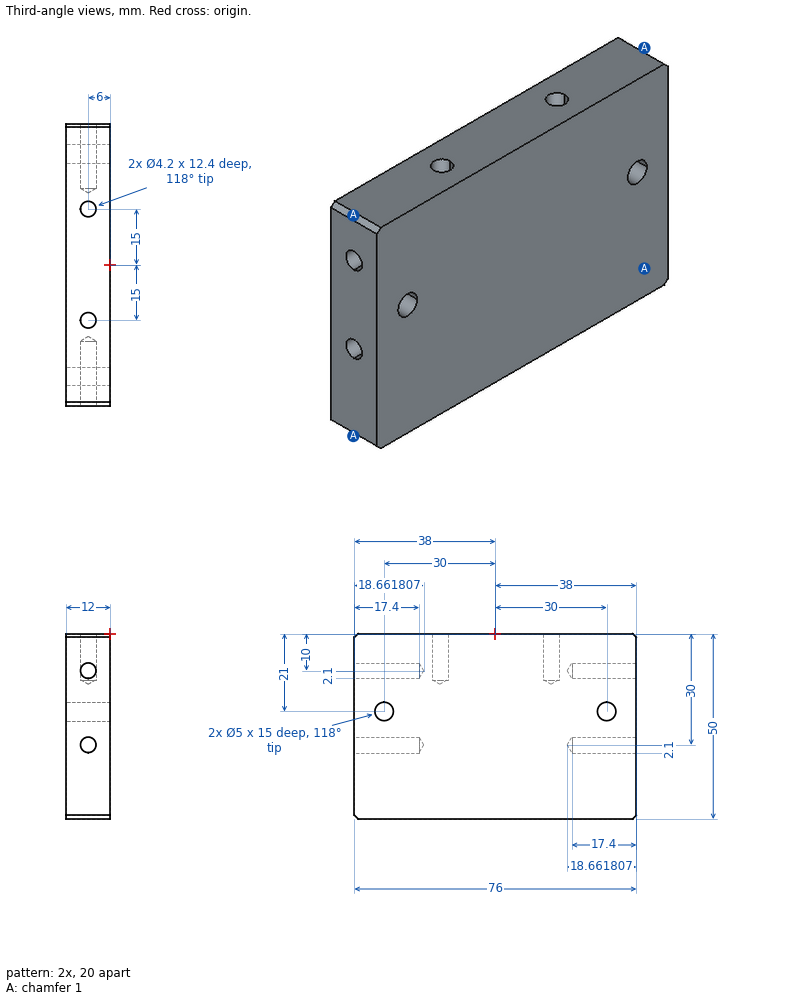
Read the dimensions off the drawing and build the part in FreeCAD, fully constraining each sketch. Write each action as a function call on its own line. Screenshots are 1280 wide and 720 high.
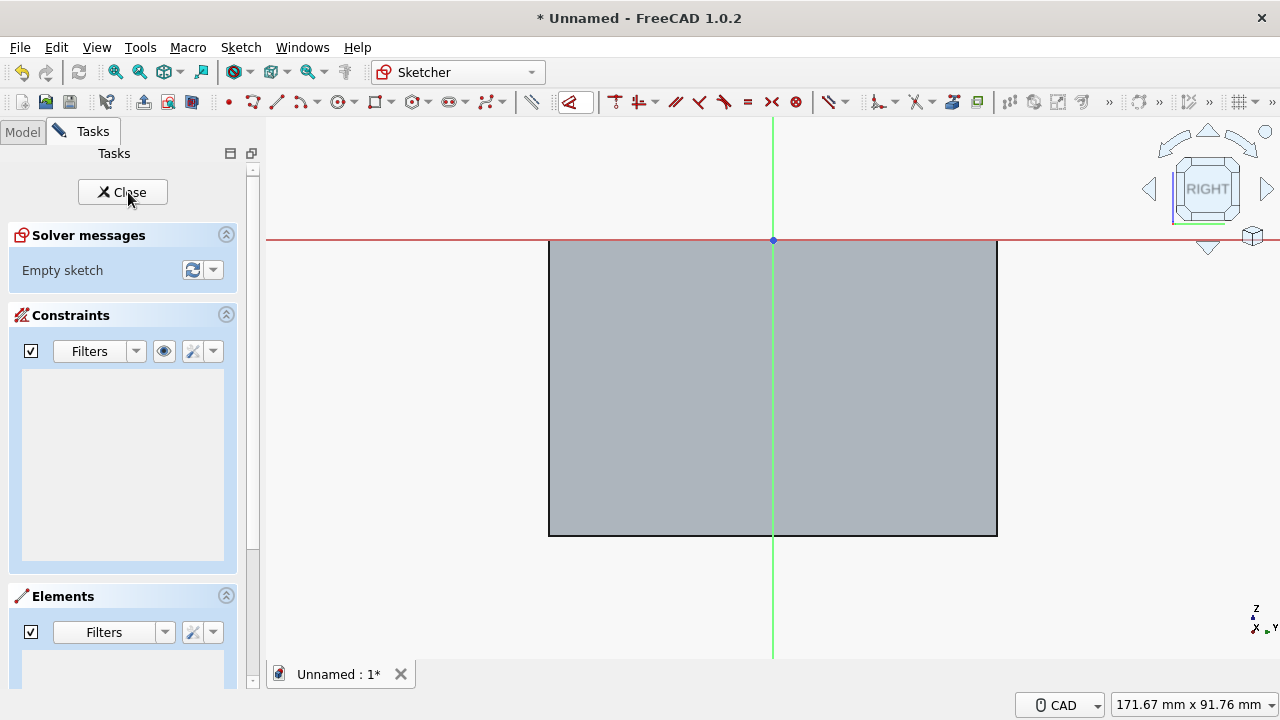
scroll(912, 151, up, 2)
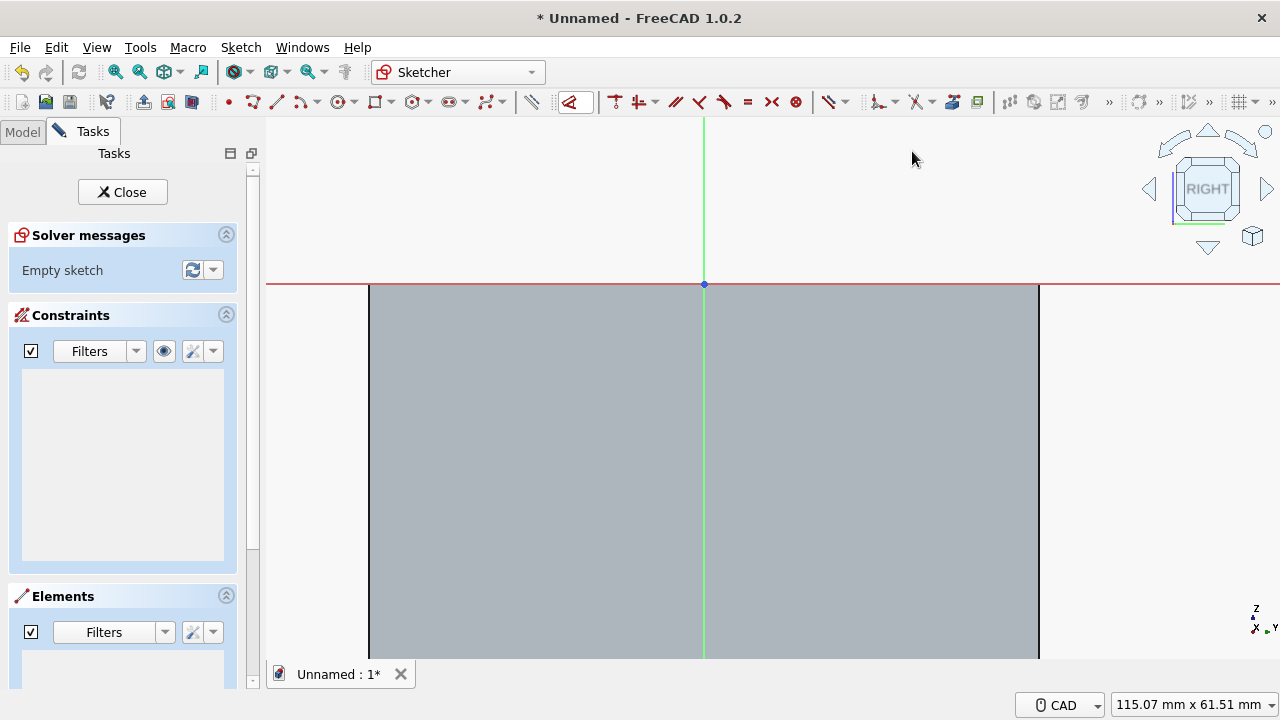
click(338, 102)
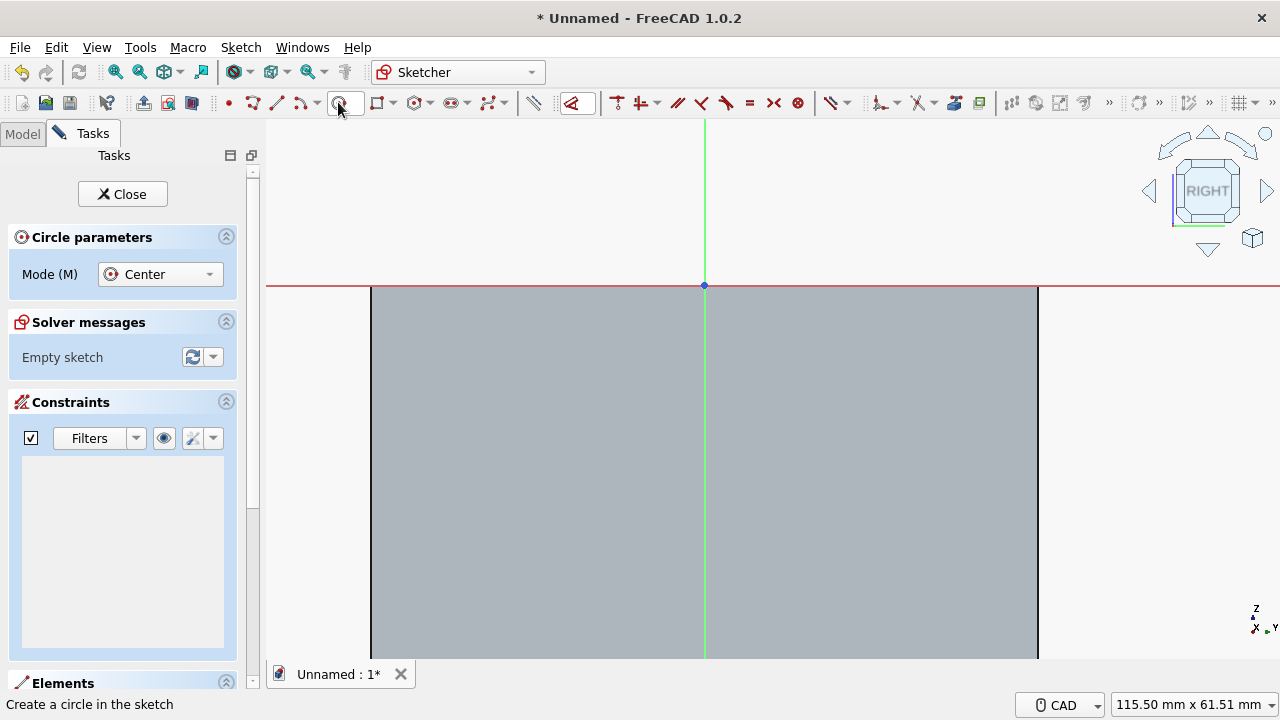
click(441, 470)
move(457, 454)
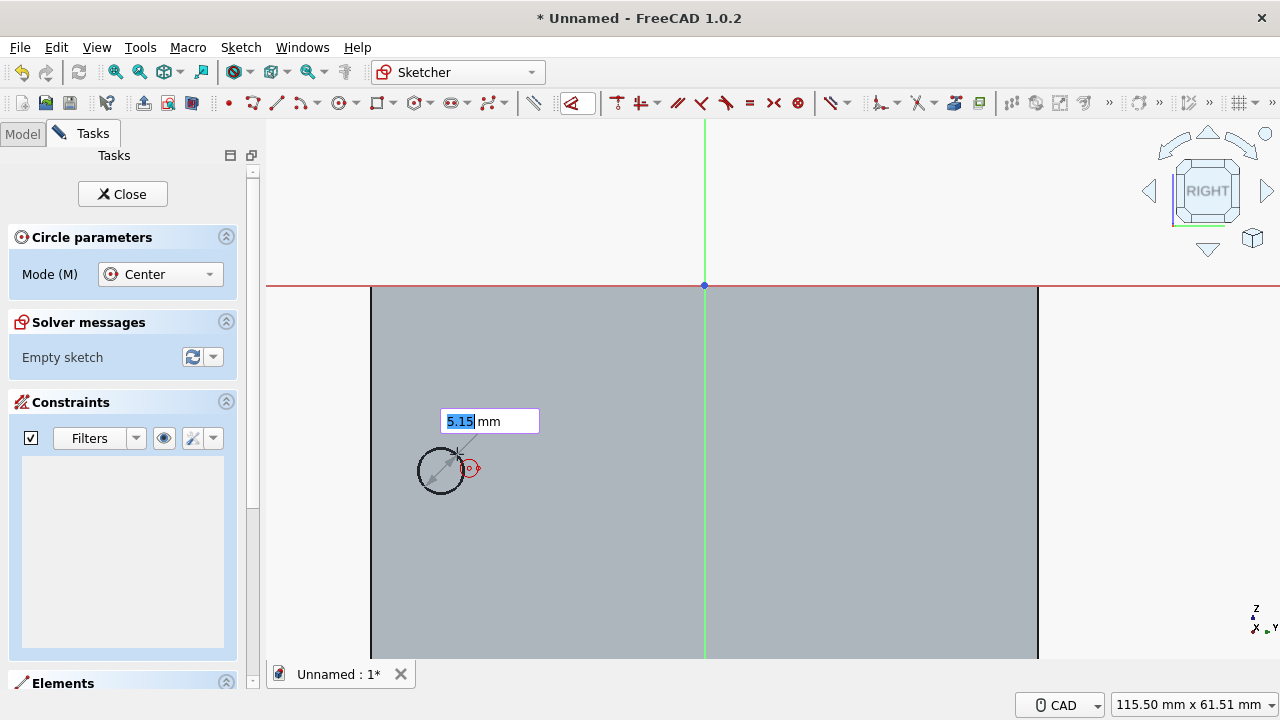
text(5)
key(Return)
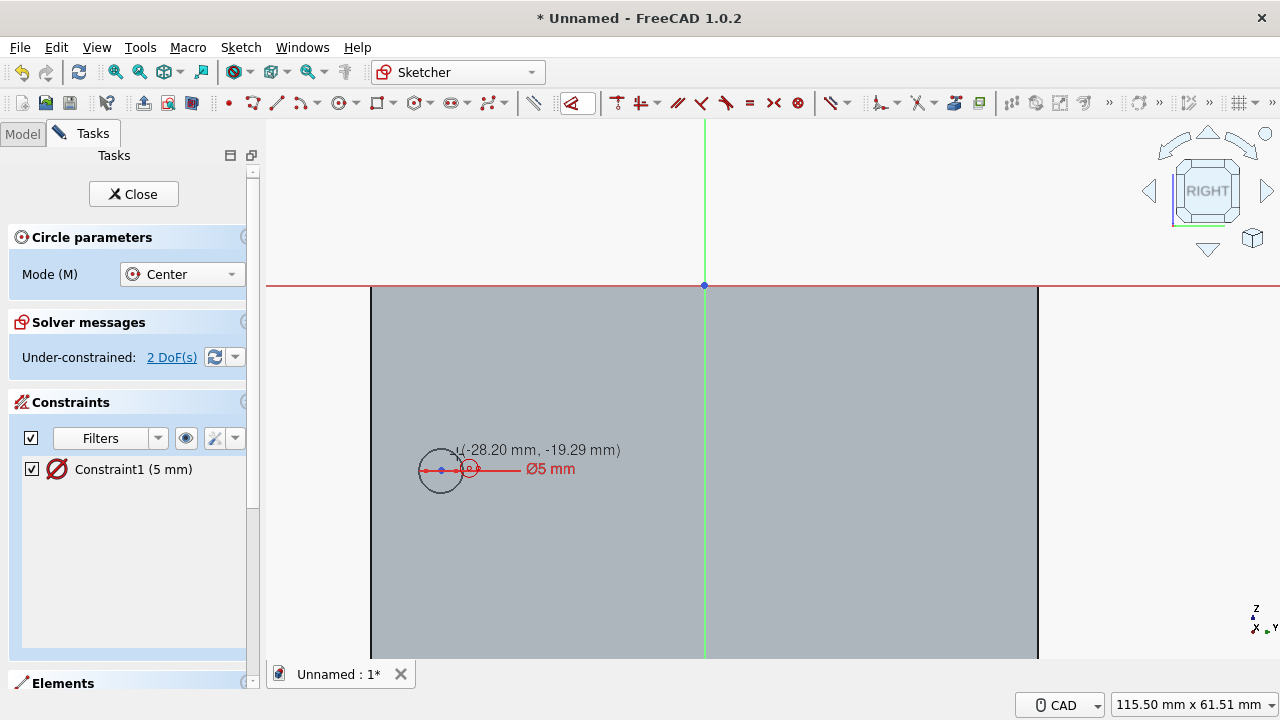
click(968, 470)
move(983, 454)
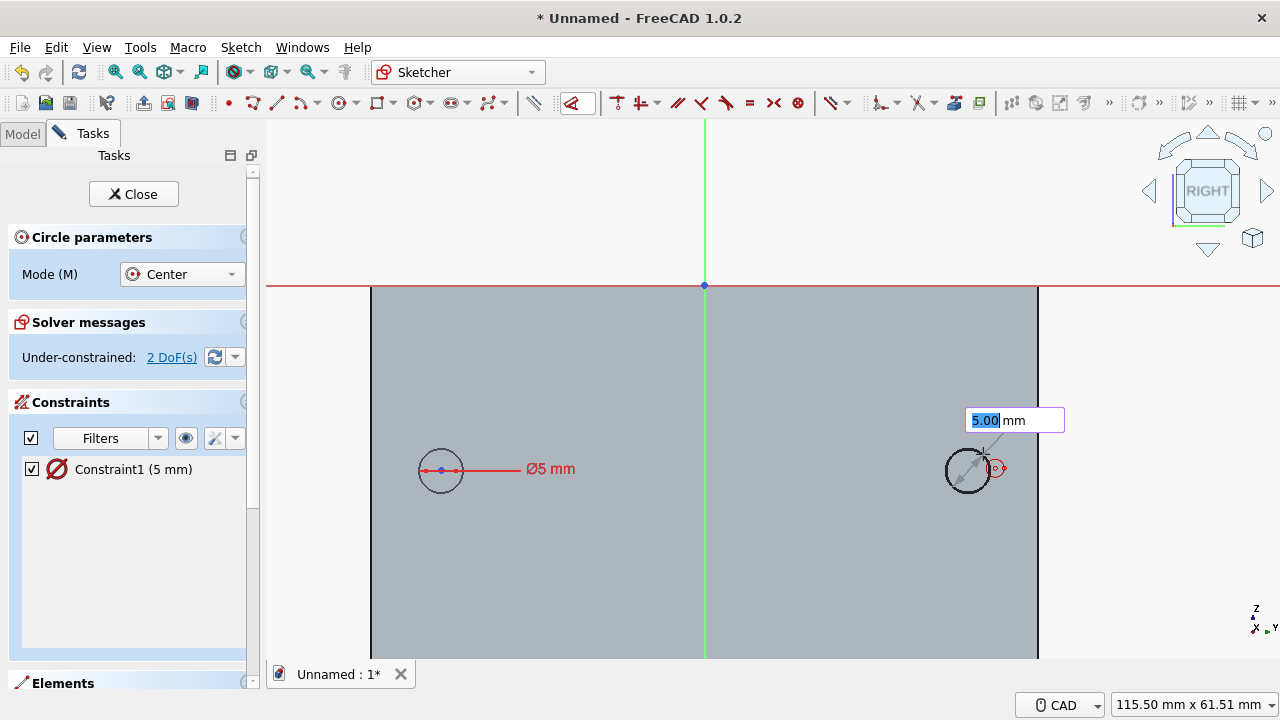
text(5)
key(Return)
key(Escape)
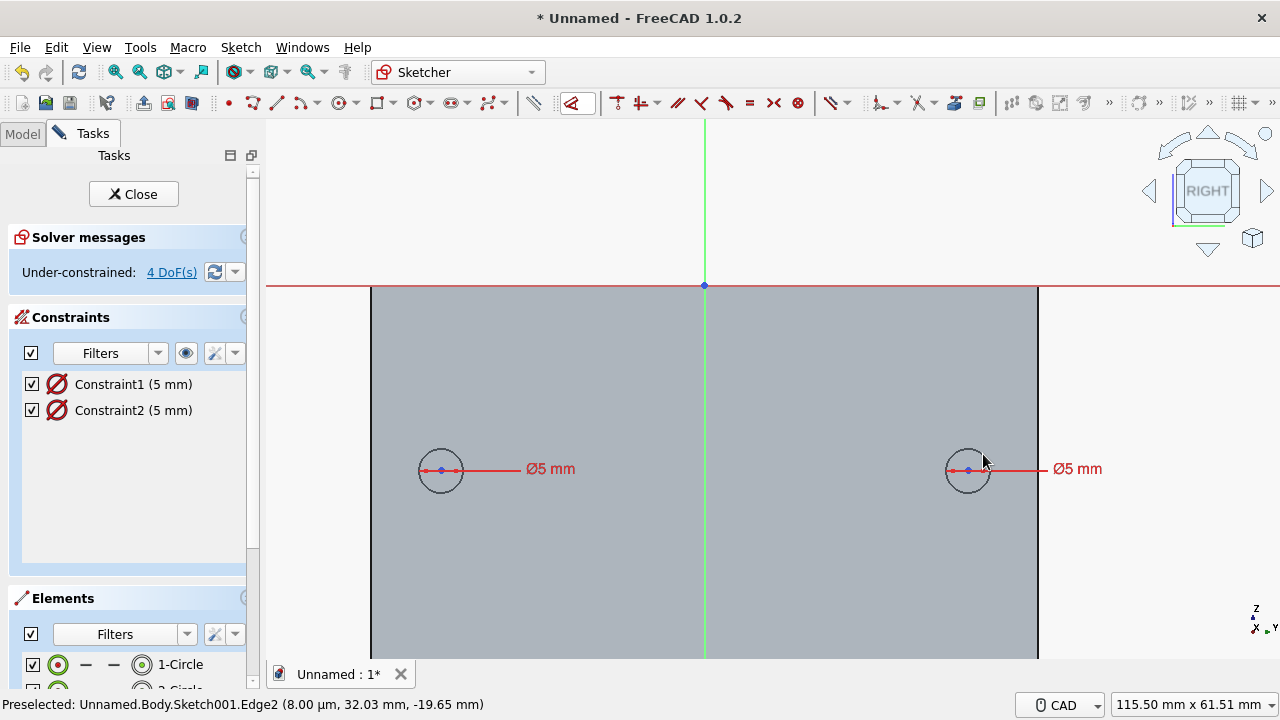
click(441, 471)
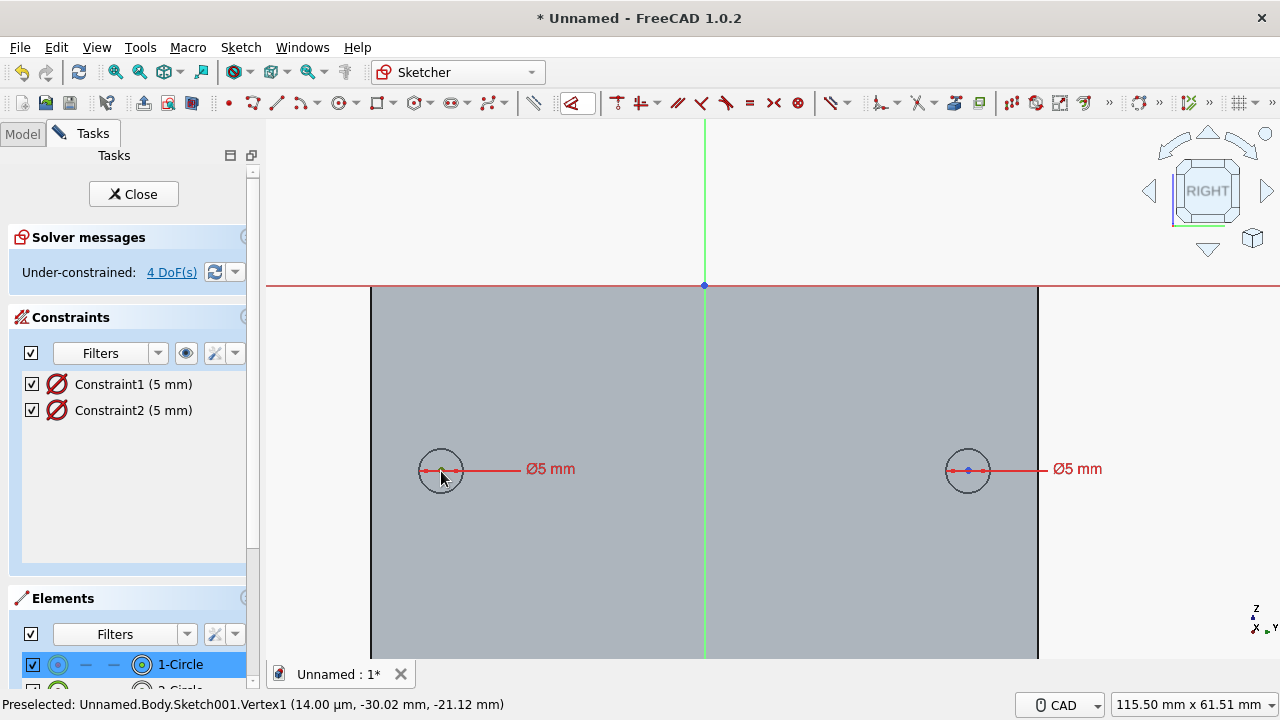
click(968, 471)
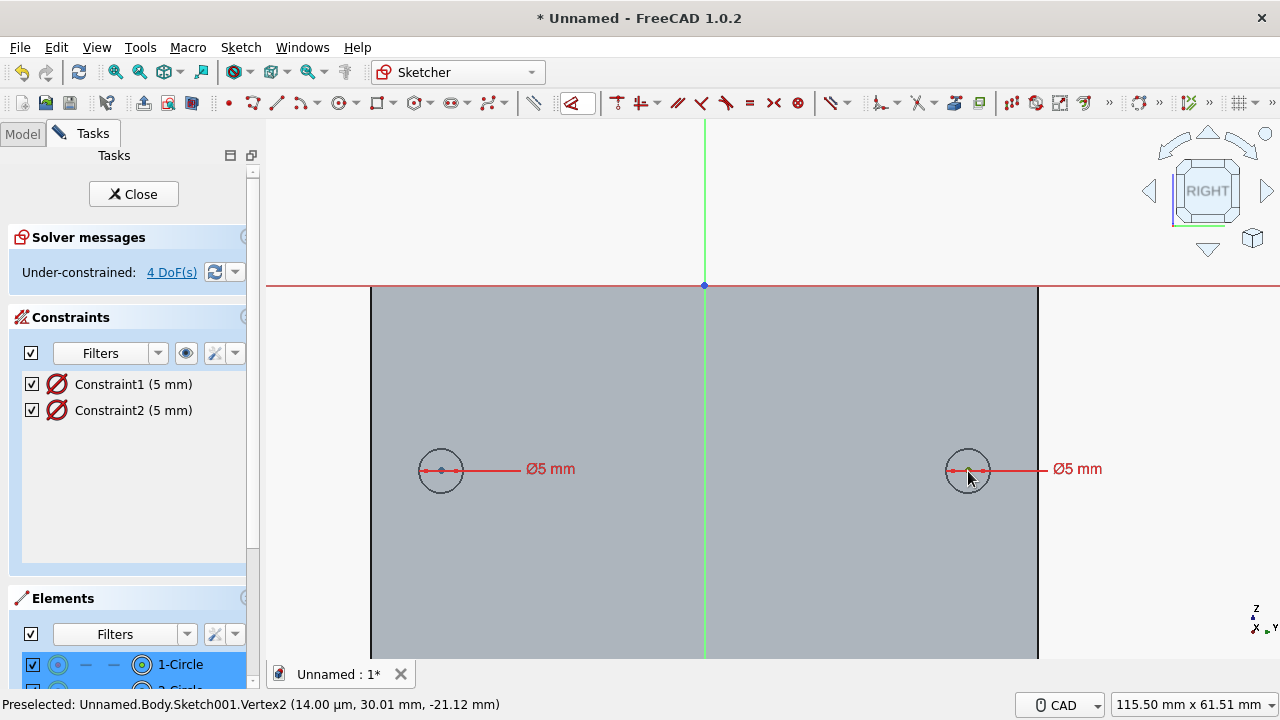
click(660, 104)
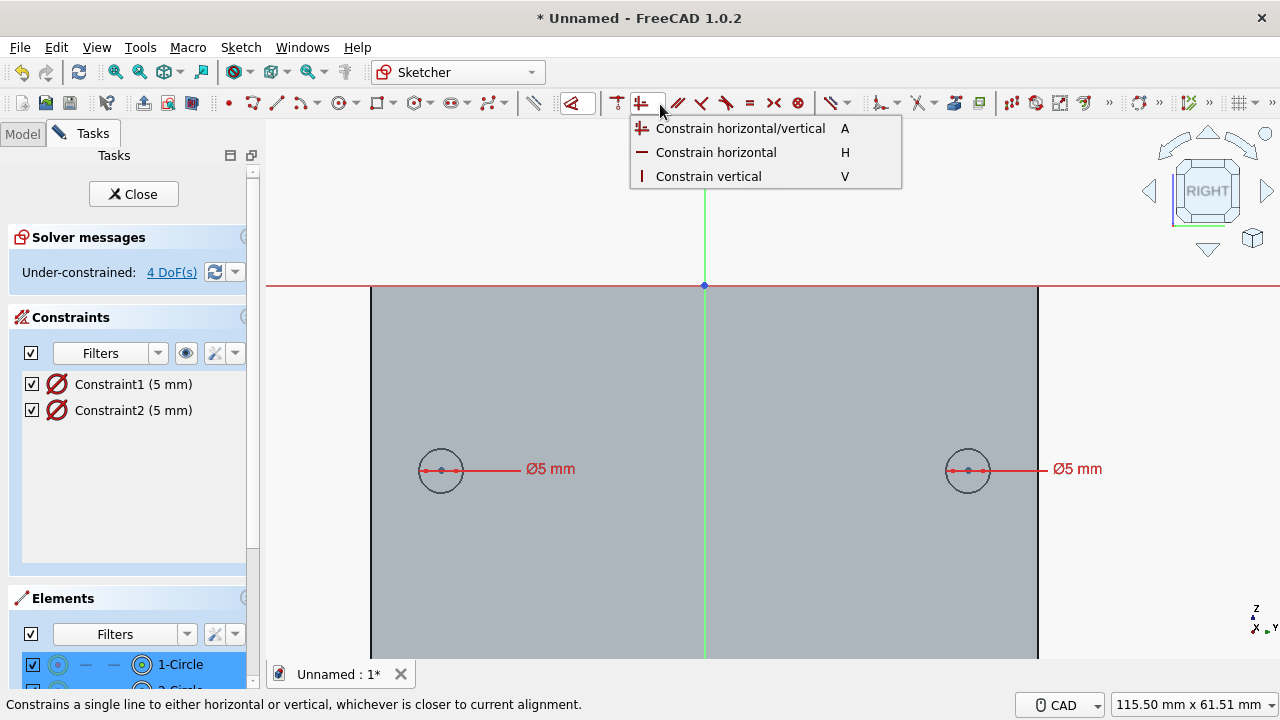
click(766, 152)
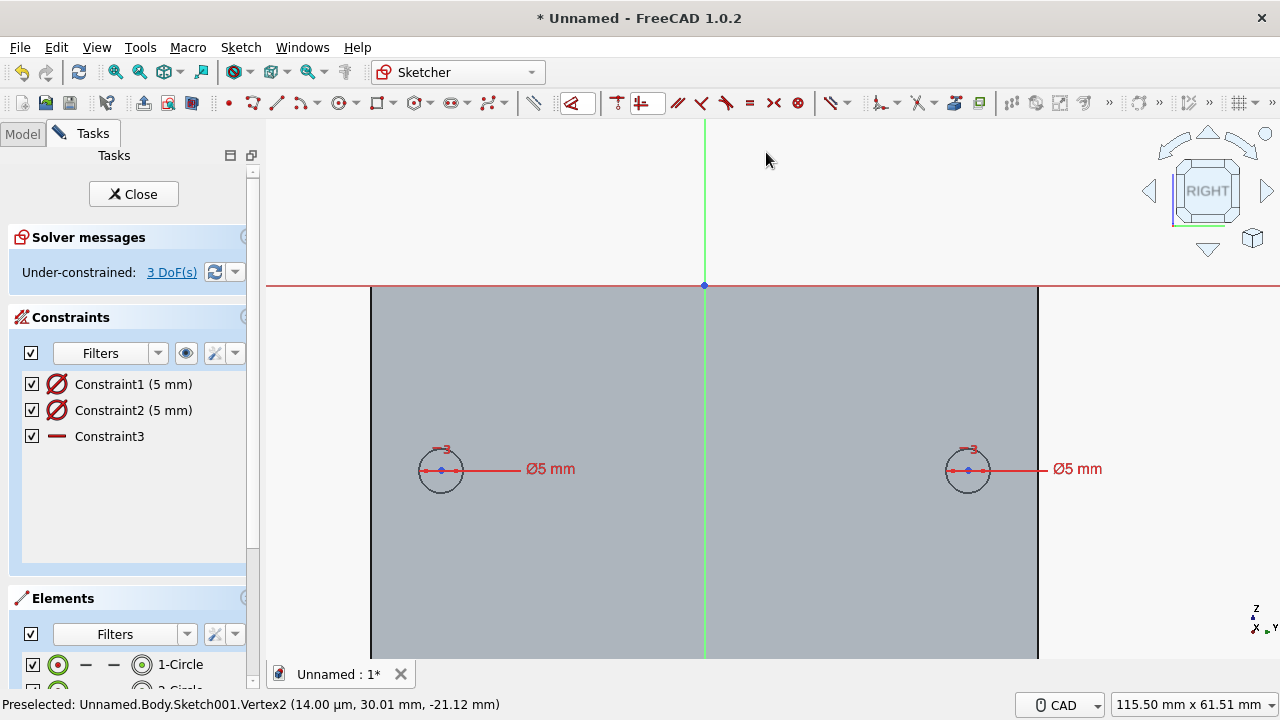
click(441, 471)